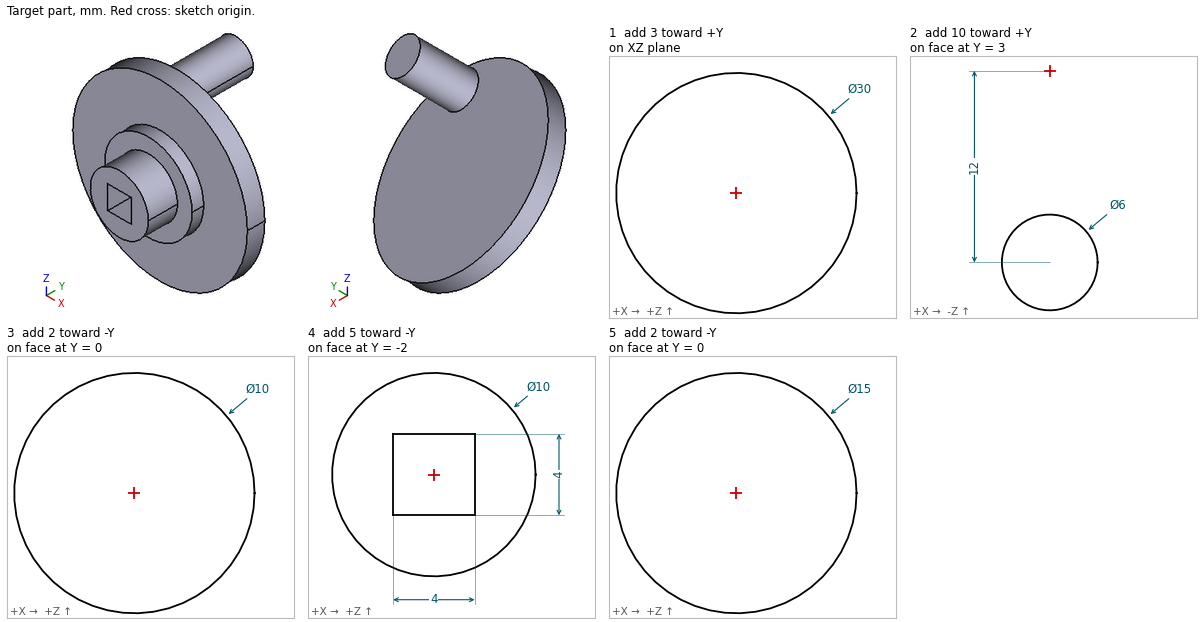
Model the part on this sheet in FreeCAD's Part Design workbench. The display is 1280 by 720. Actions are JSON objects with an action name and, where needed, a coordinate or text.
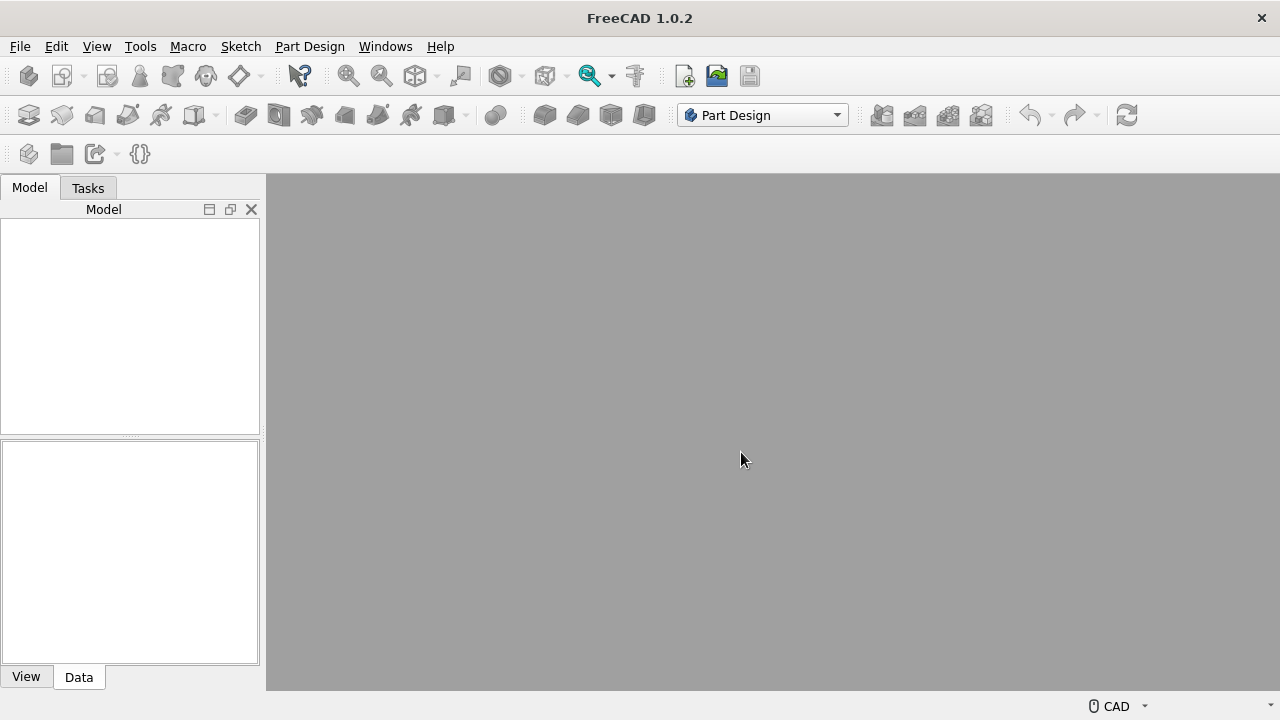
{"action": "left_click", "coordinate": [684, 76]}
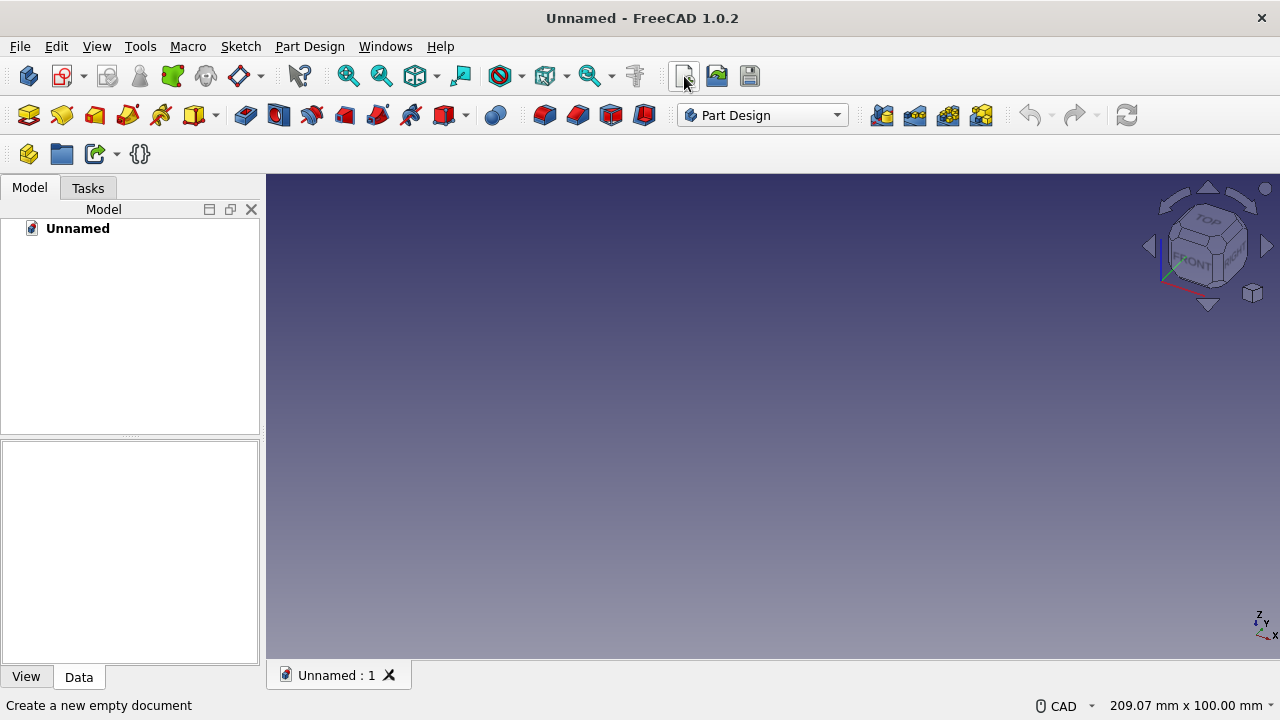
{"action": "left_click", "coordinate": [62, 76]}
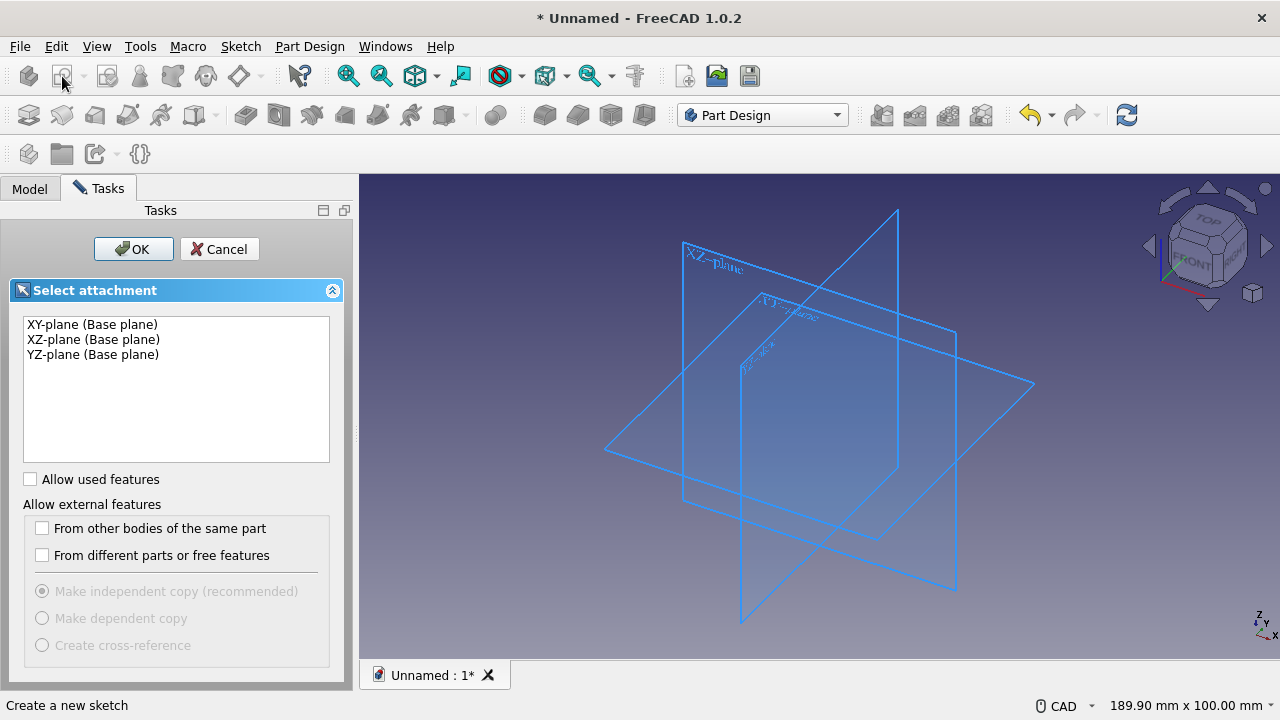
{"action": "left_click", "coordinate": [84, 340]}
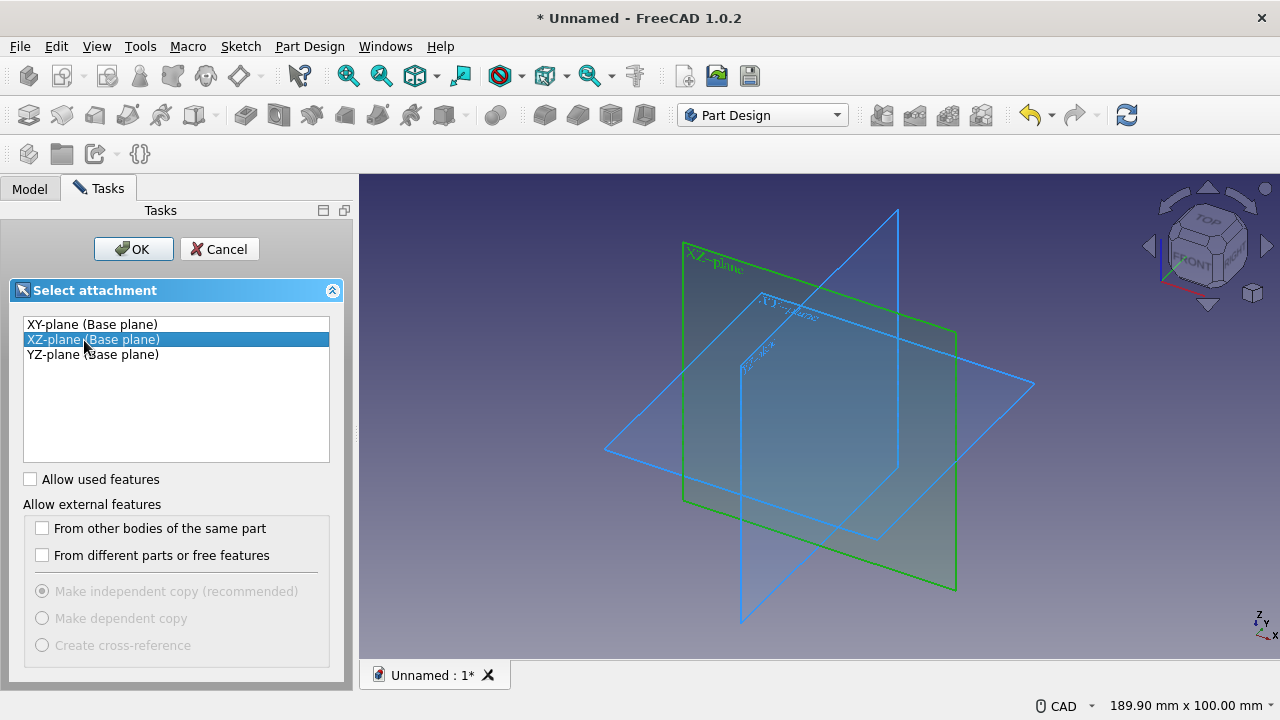
{"action": "left_click", "coordinate": [134, 249]}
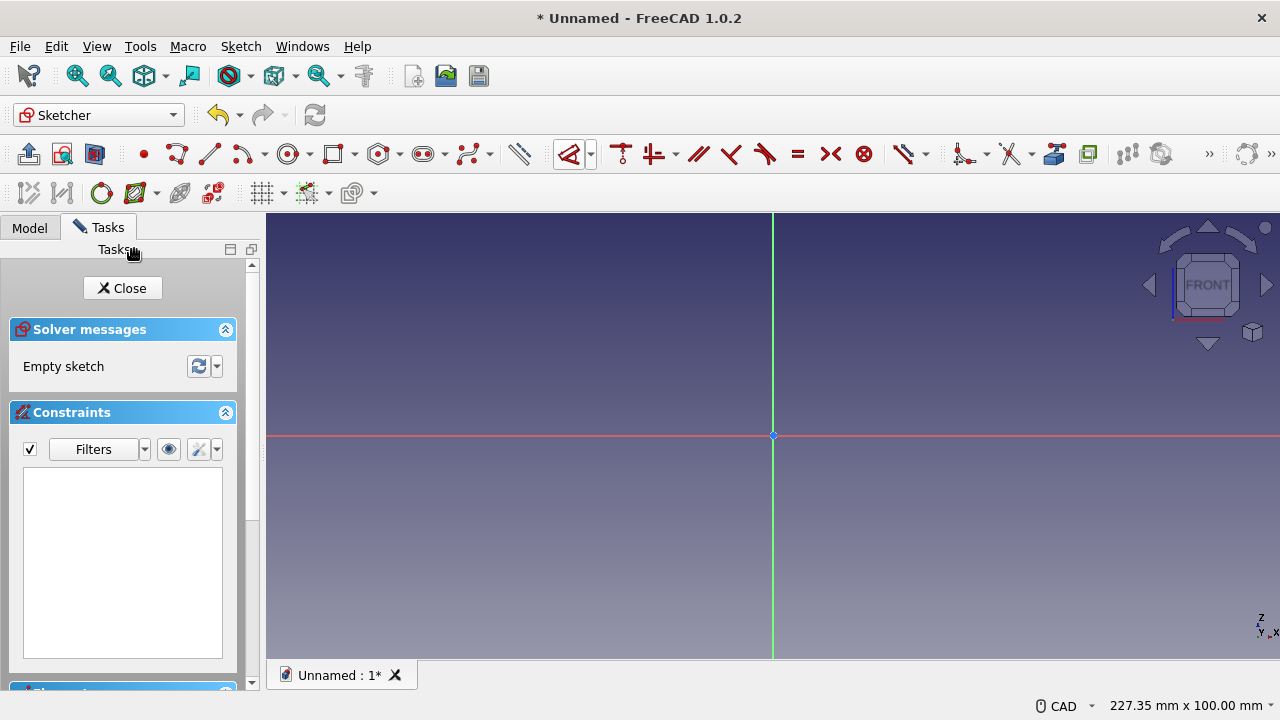
{"action": "scroll", "coordinate": [829, 436], "scroll_direction": "up", "scroll_amount": 4}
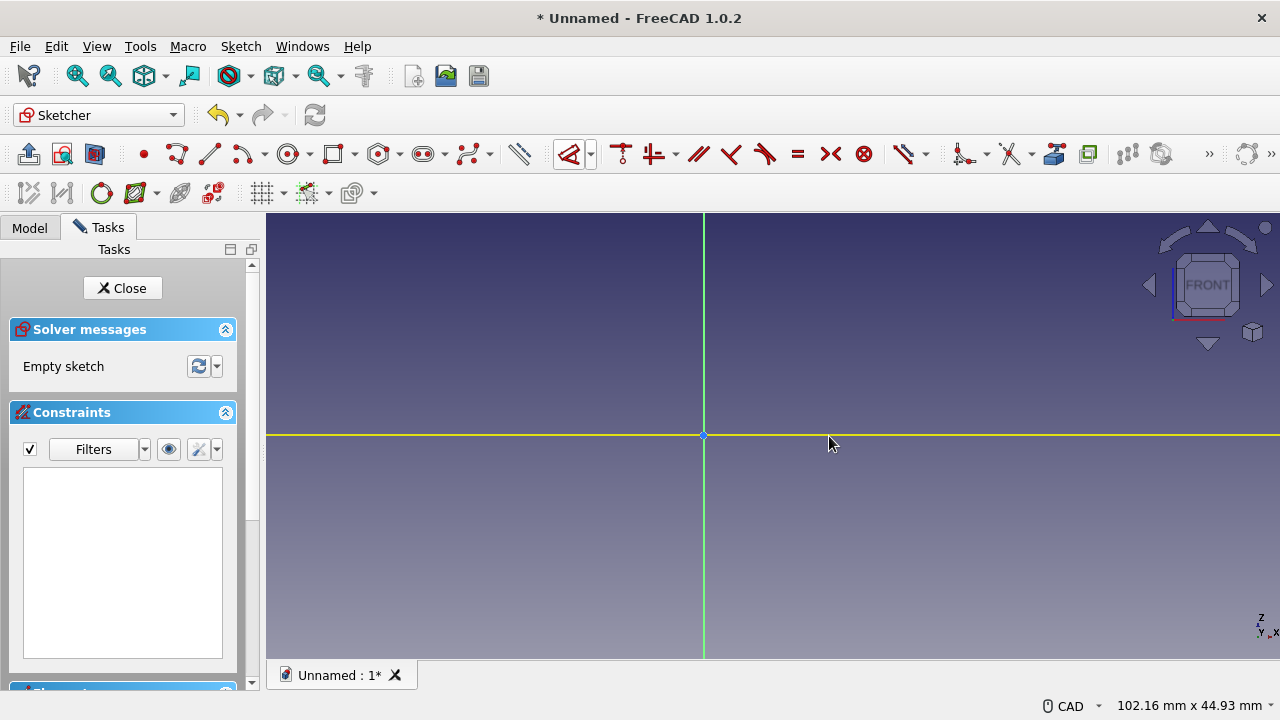
{"action": "key", "text": "g c"}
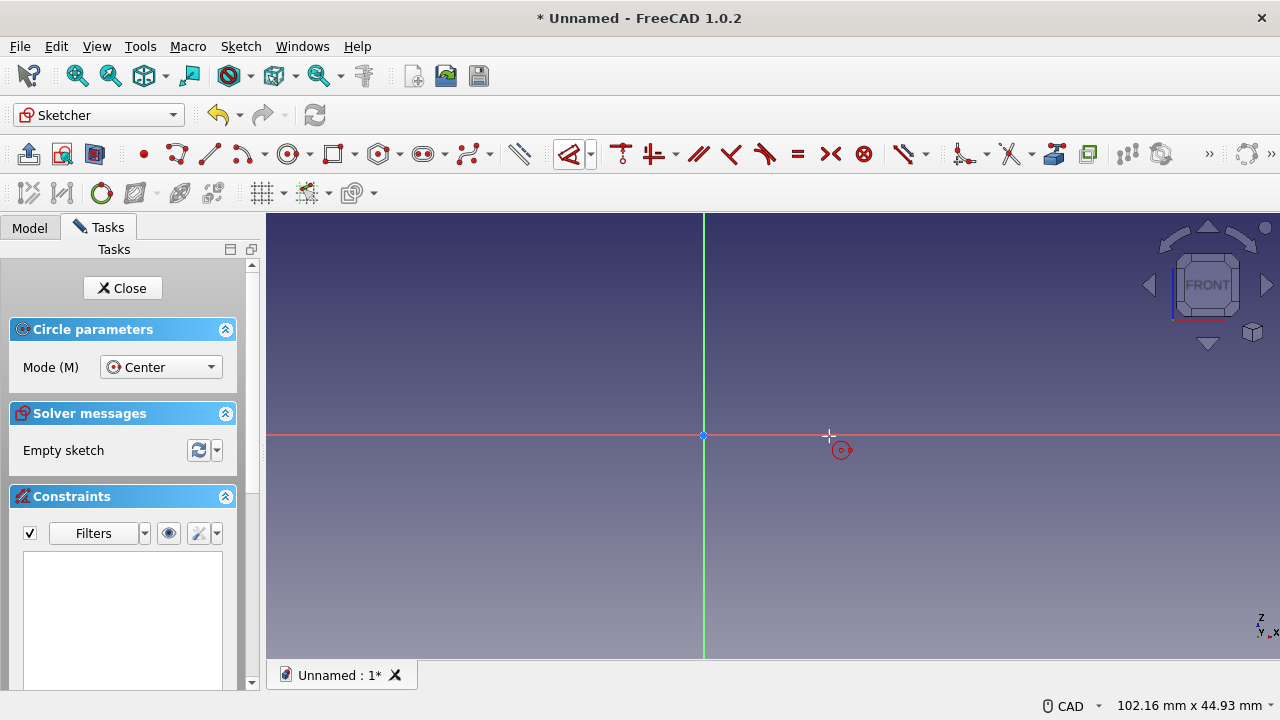
{"action": "left_click", "coordinate": [704, 435]}
{"action": "left_click", "coordinate": [809, 330]}
{"action": "key", "text": "Escape"}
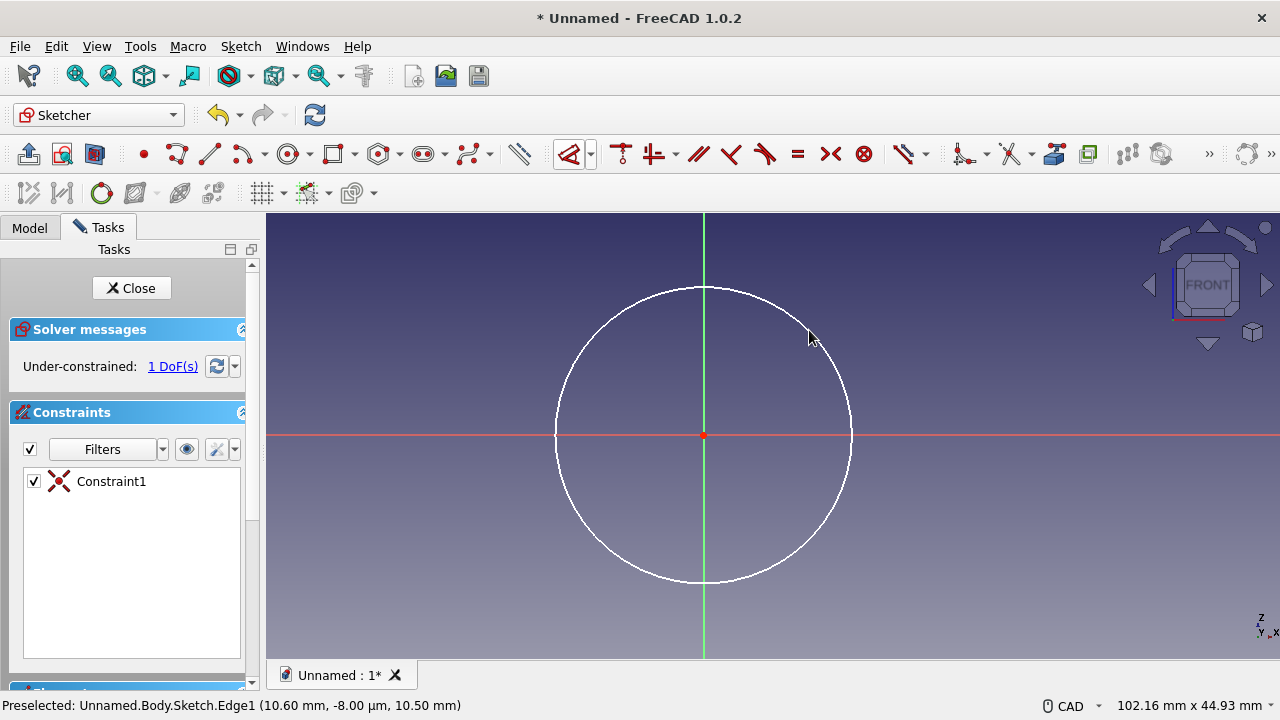
{"action": "key", "text": "d"}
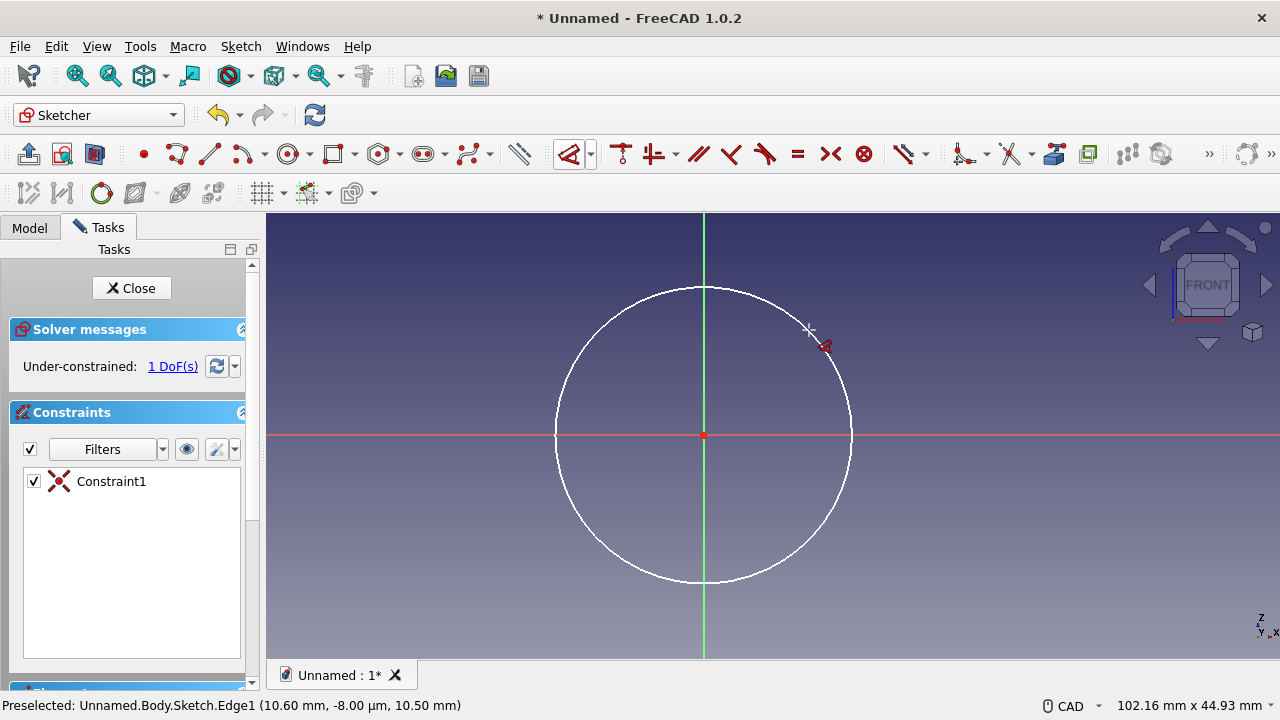
{"action": "left_click", "coordinate": [808, 330]}
{"action": "left_click", "coordinate": [831, 307]}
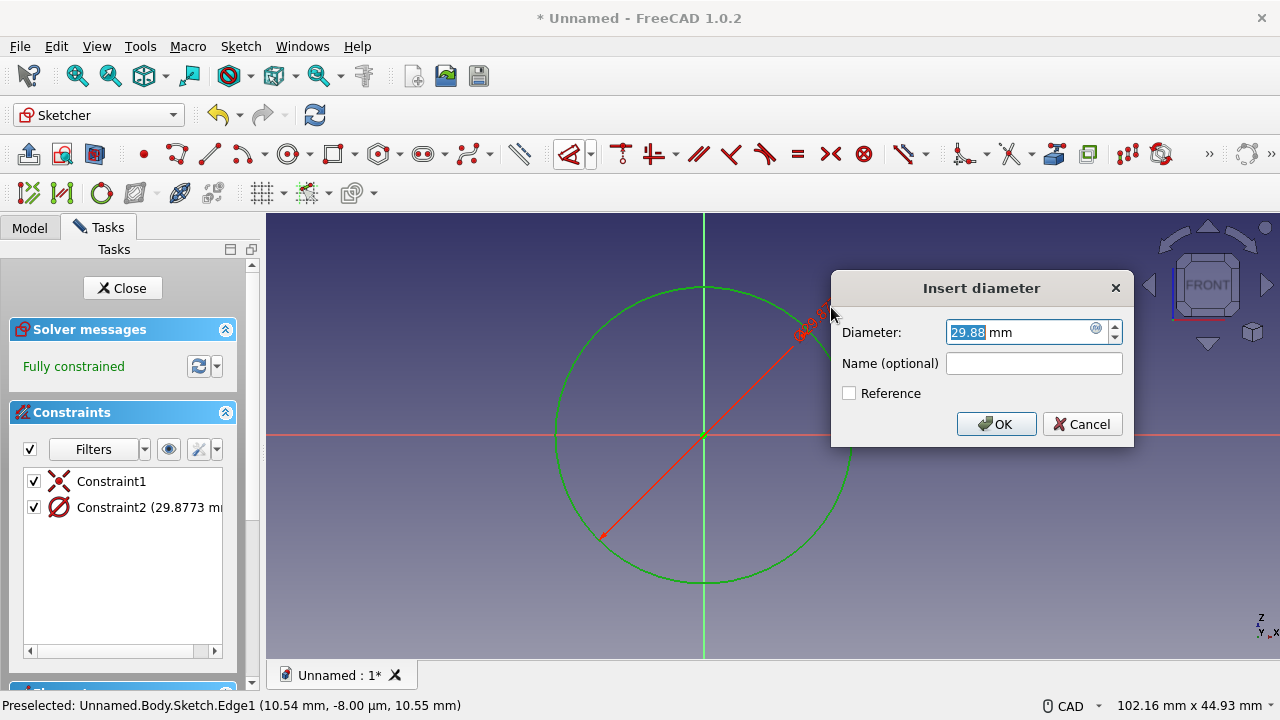
{"action": "type", "text": "30"}
{"action": "key", "text": "Return"}
{"action": "key", "text": "Escape"}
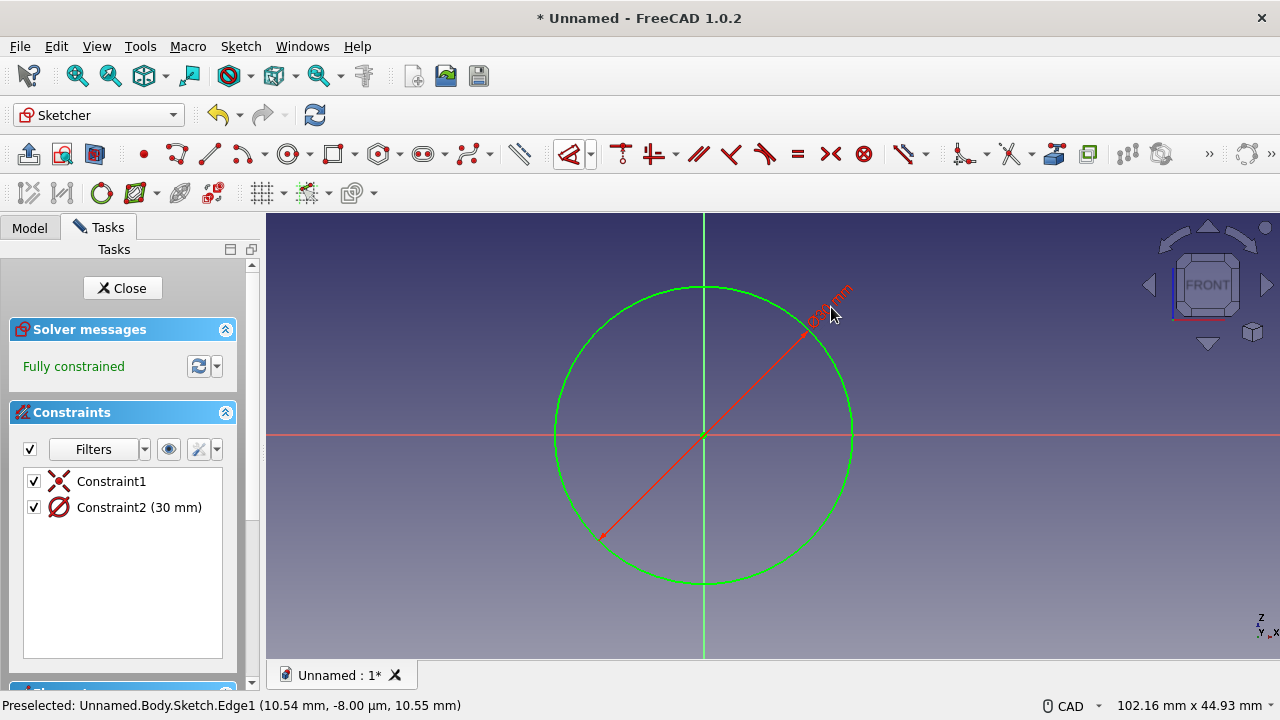
{"action": "left_click", "coordinate": [123, 288]}